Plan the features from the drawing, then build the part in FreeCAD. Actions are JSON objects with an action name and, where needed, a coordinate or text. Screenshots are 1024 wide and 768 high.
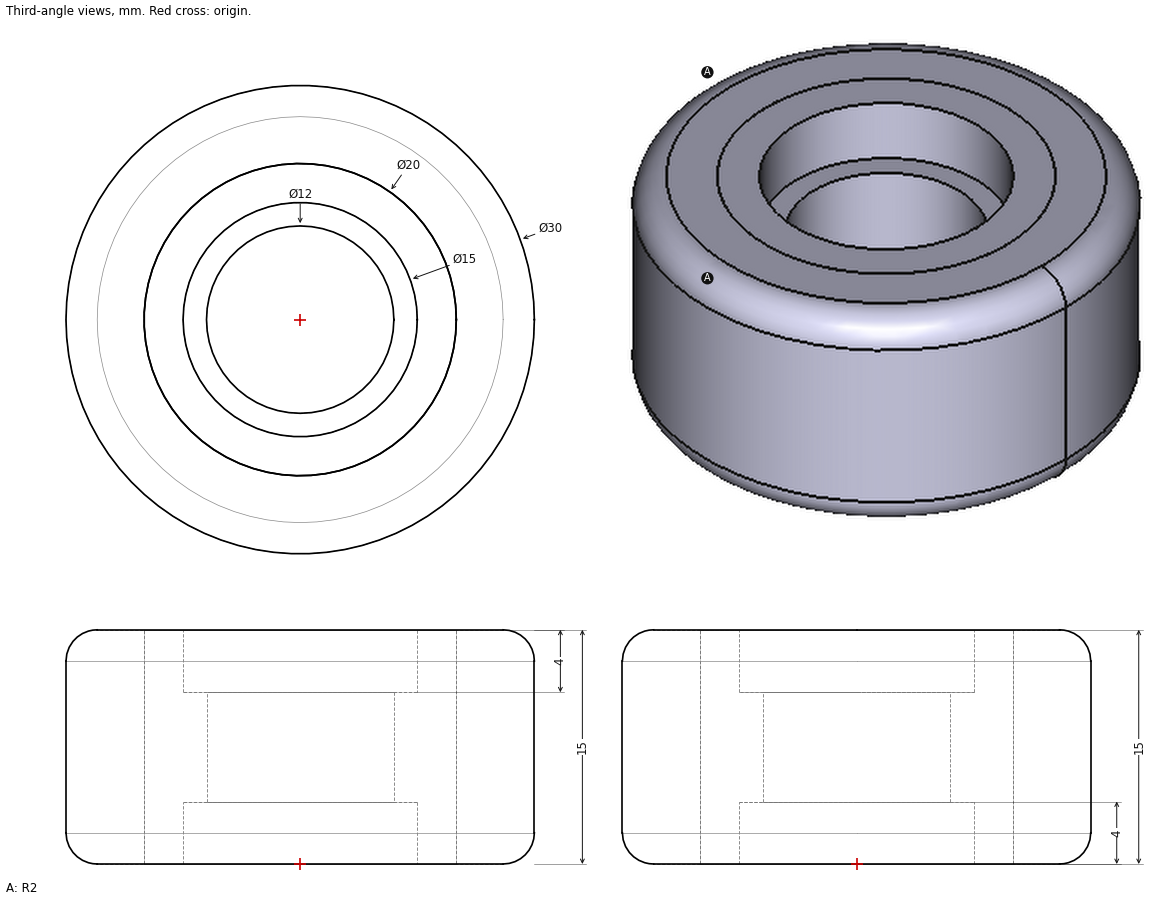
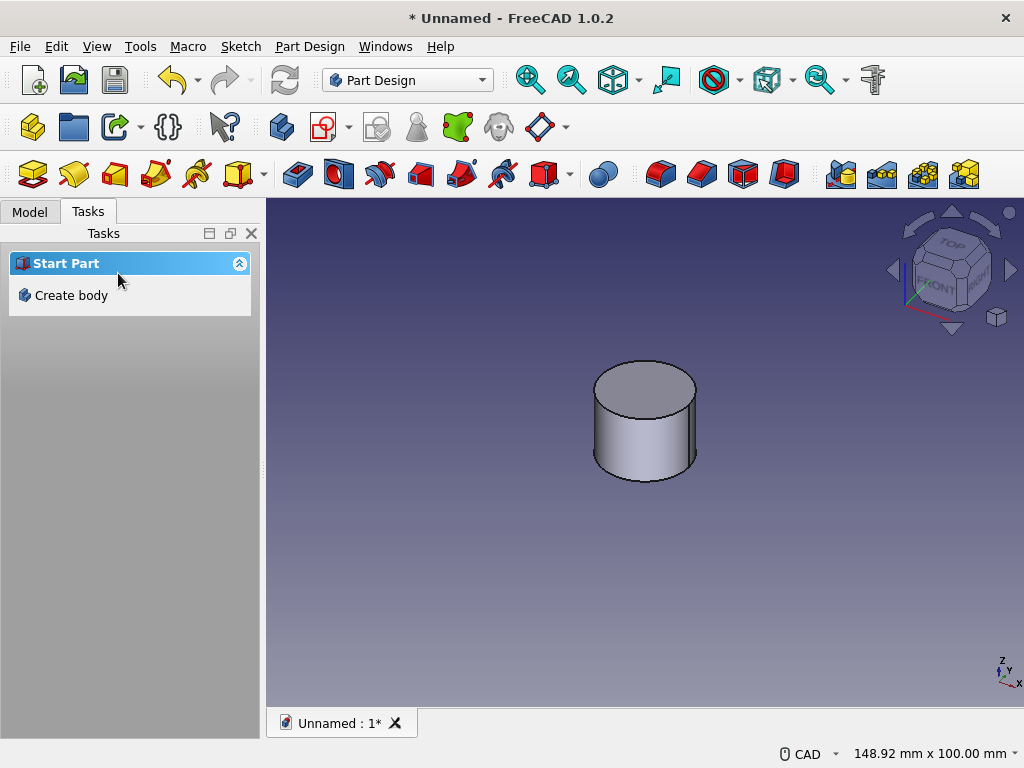
{"action": "key", "text": "v f"}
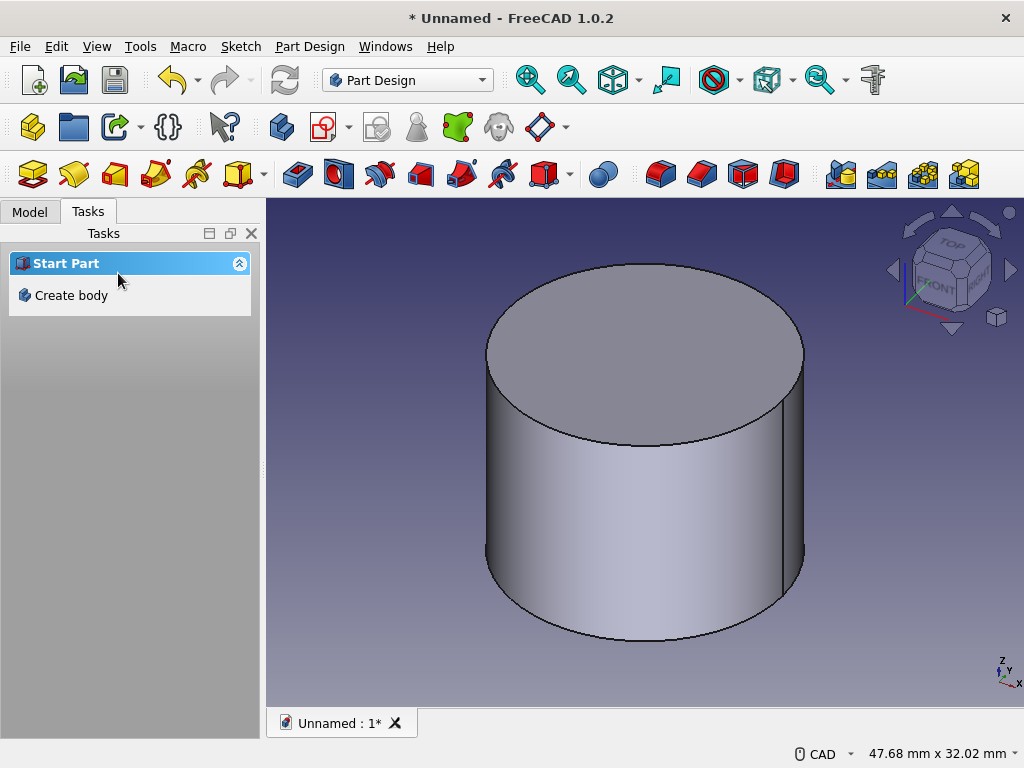
{"action": "left_click", "coordinate": [645, 354]}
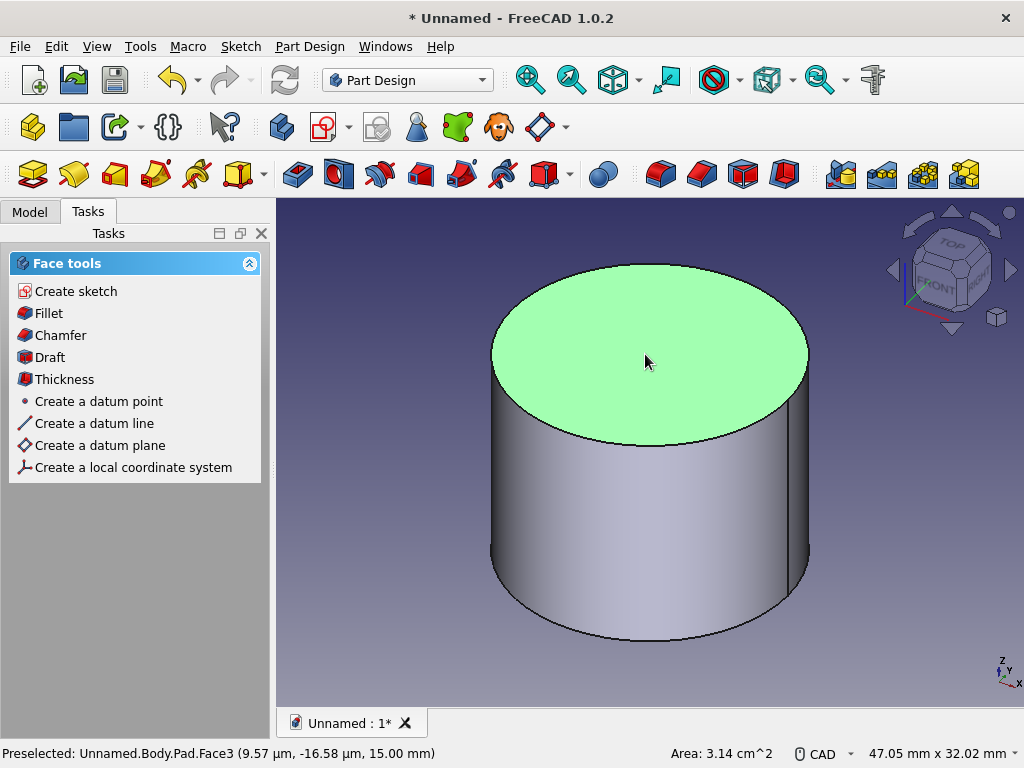
{"action": "left_click", "coordinate": [322, 128]}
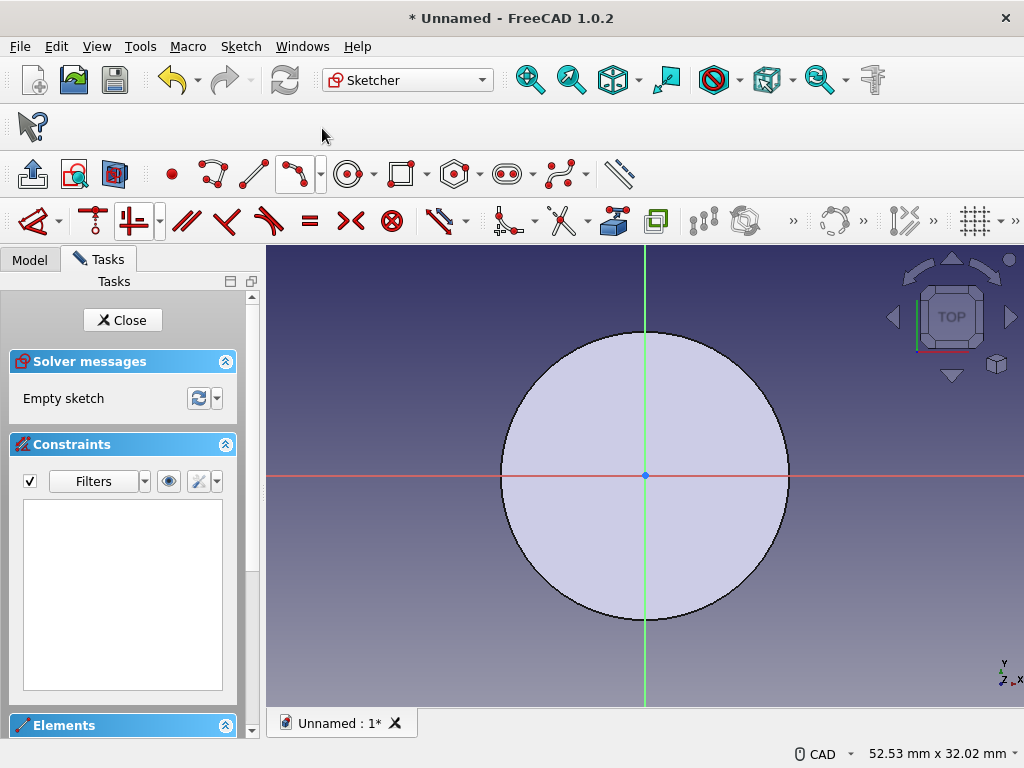
{"action": "scroll", "coordinate": [728, 476], "scroll_direction": "up", "scroll_amount": 3}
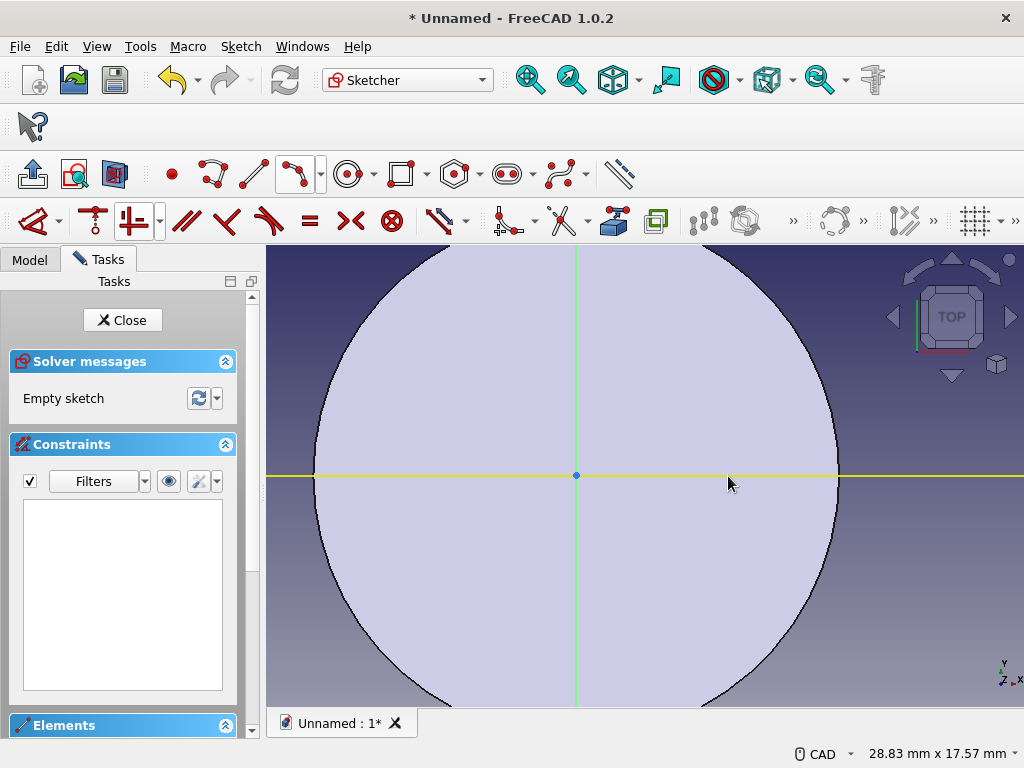
{"action": "key", "text": "g c"}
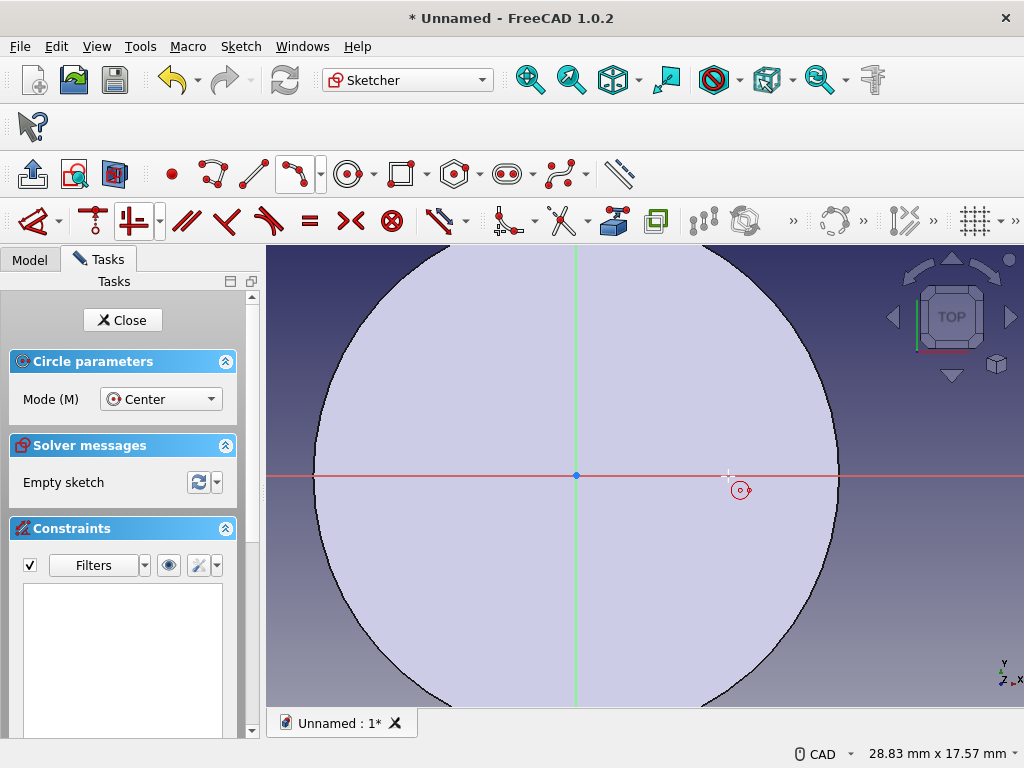
{"action": "left_click", "coordinate": [576, 476]}
{"action": "mouse_move", "coordinate": [688, 364]}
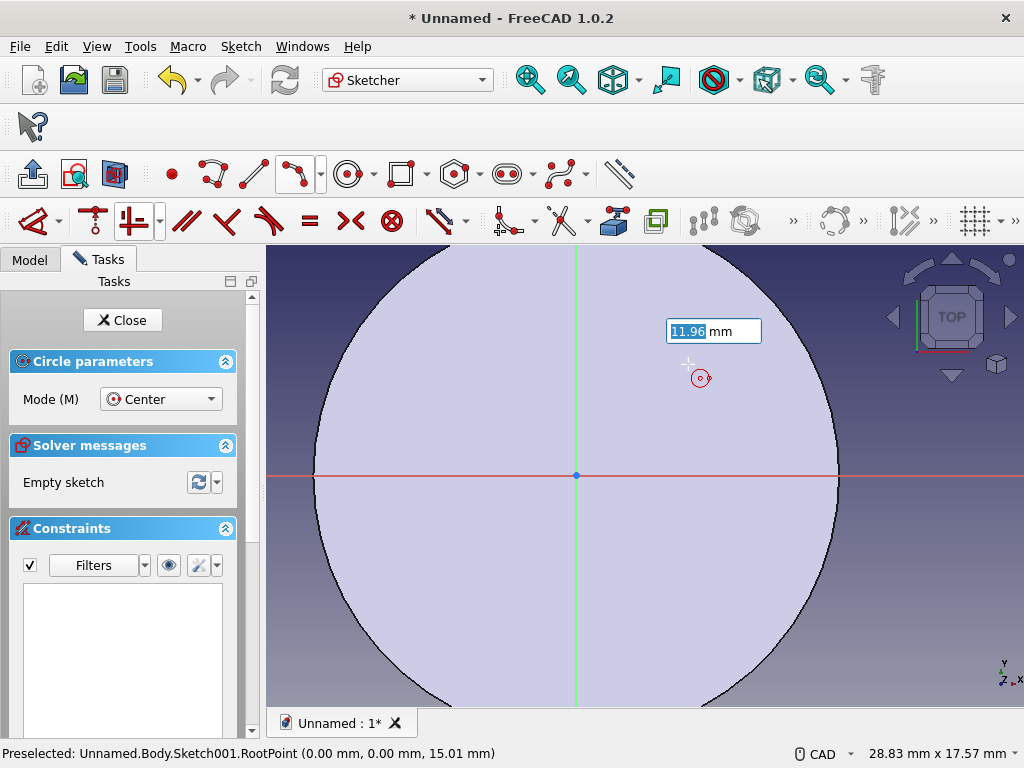
{"action": "type", "text": "12"}
{"action": "key", "text": "Return"}
{"action": "key", "text": "Escape"}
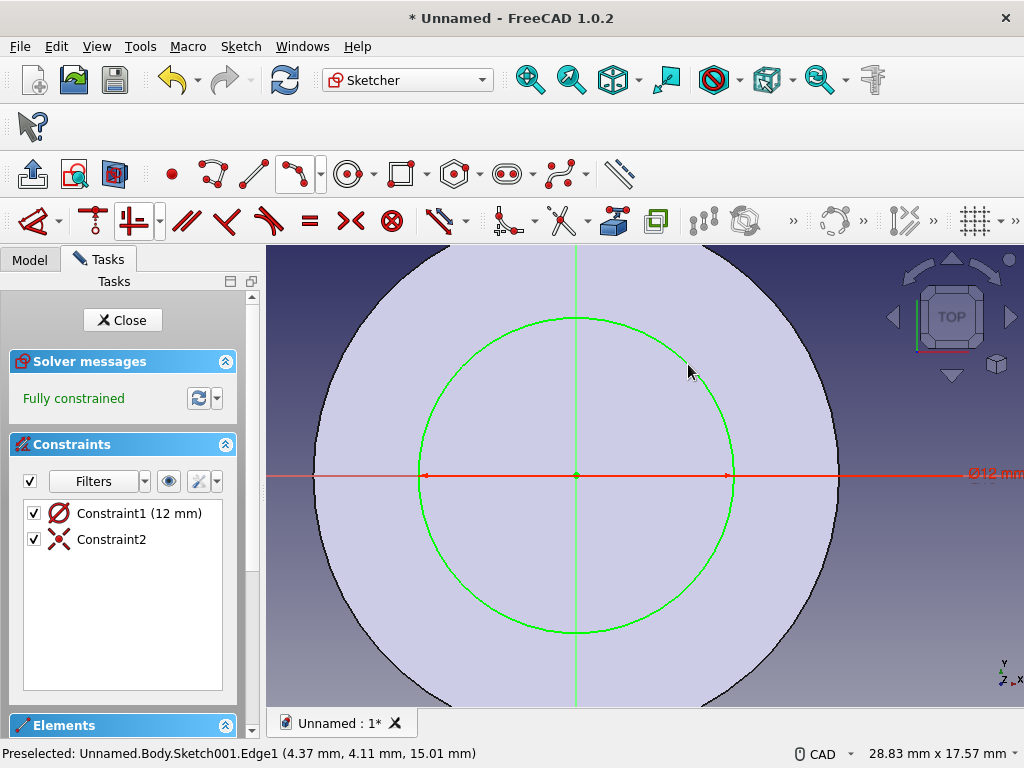
{"action": "left_click", "coordinate": [123, 320]}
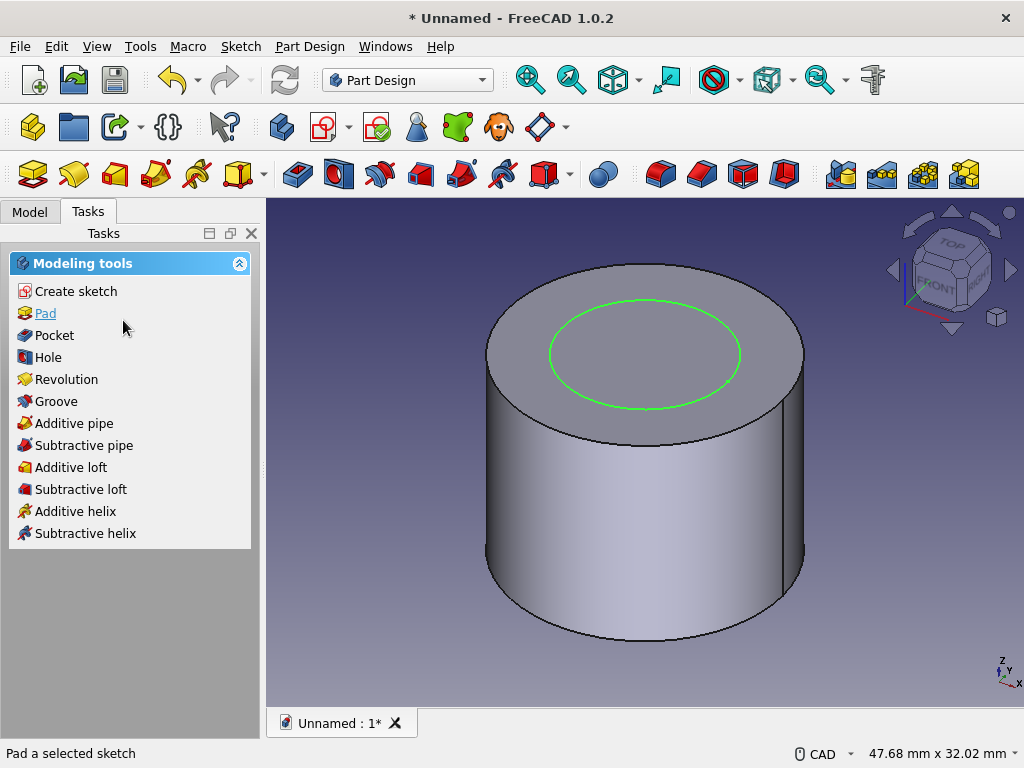
{"action": "left_click", "coordinate": [298, 174]}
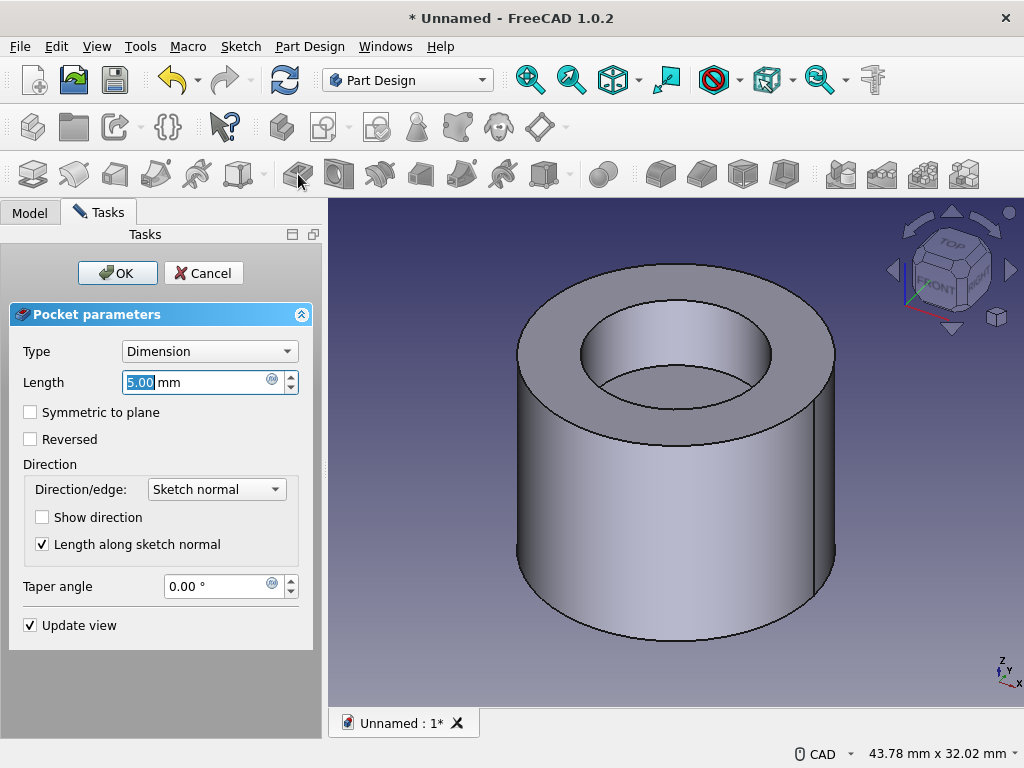
{"action": "left_click", "coordinate": [210, 352]}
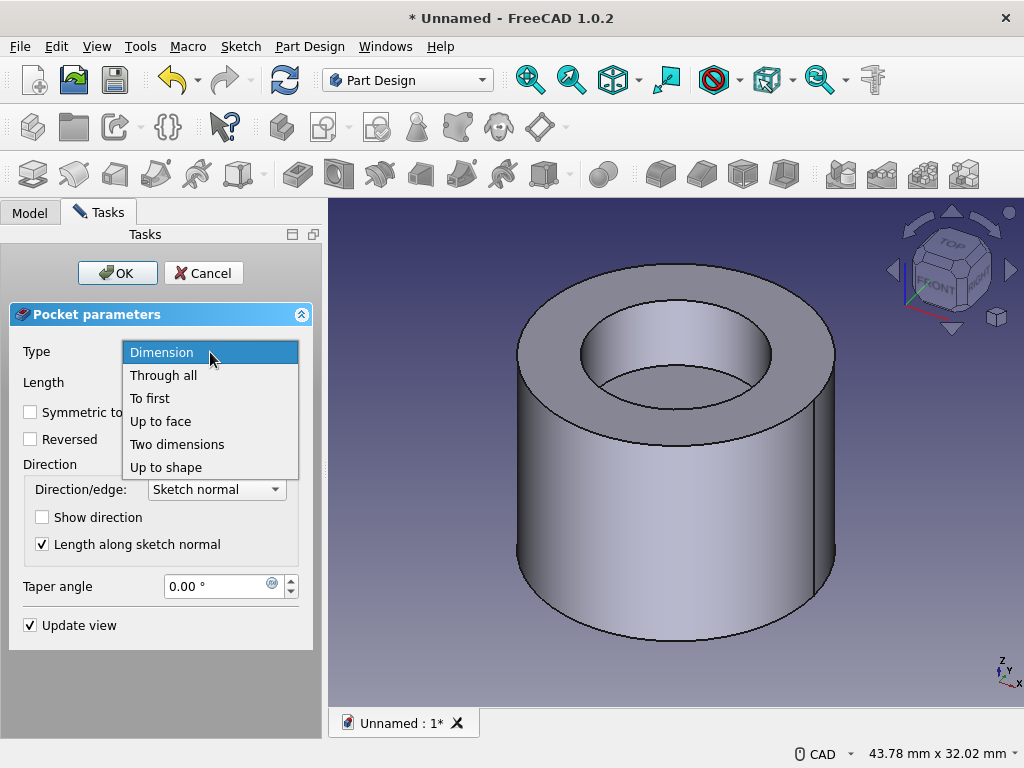
{"action": "left_click", "coordinate": [208, 376]}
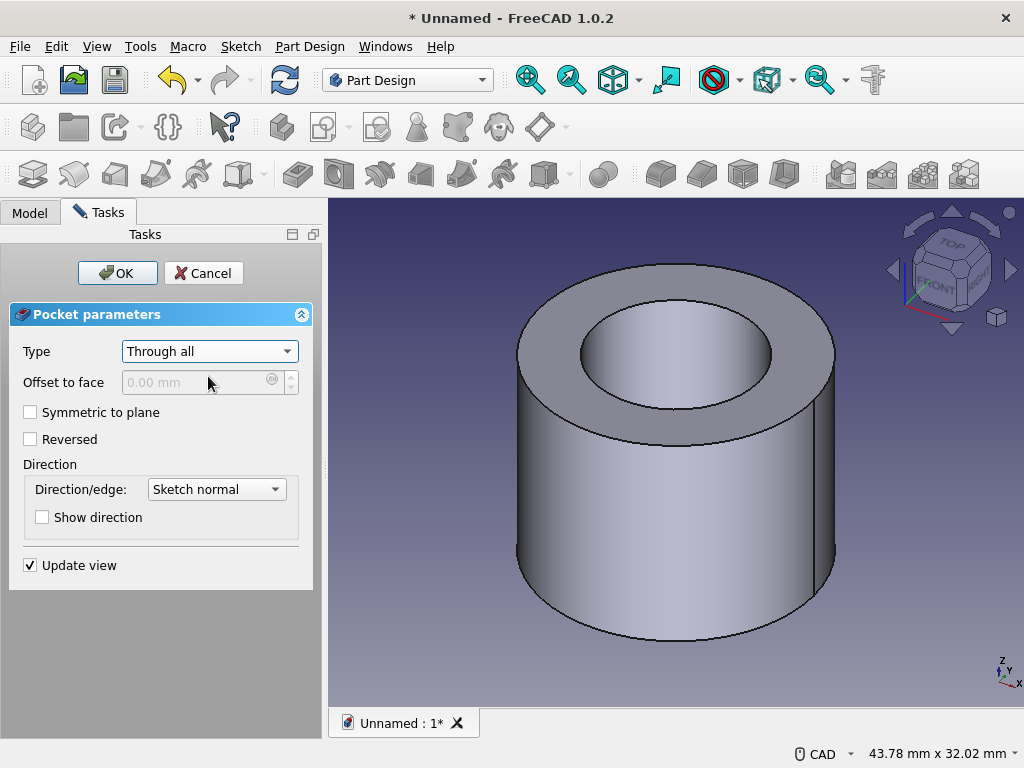
{"action": "left_click", "coordinate": [118, 273]}